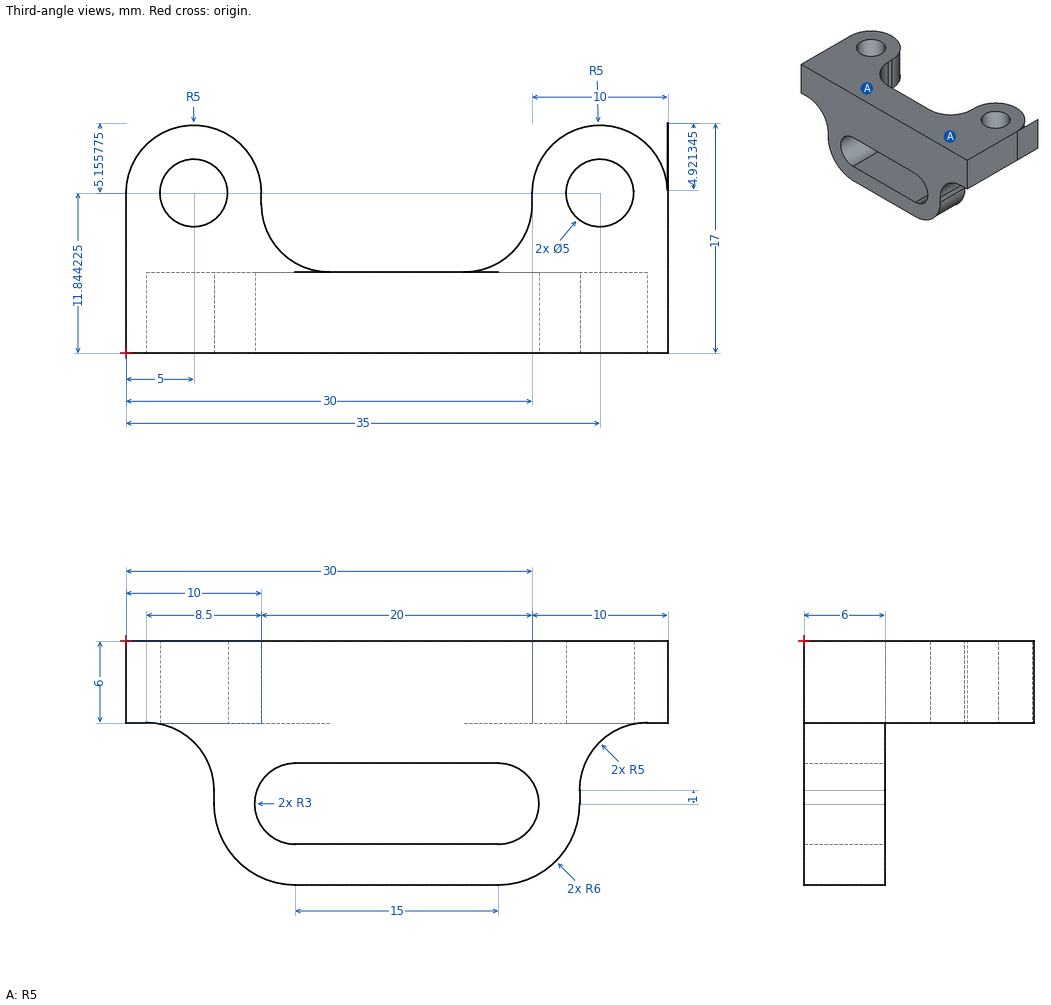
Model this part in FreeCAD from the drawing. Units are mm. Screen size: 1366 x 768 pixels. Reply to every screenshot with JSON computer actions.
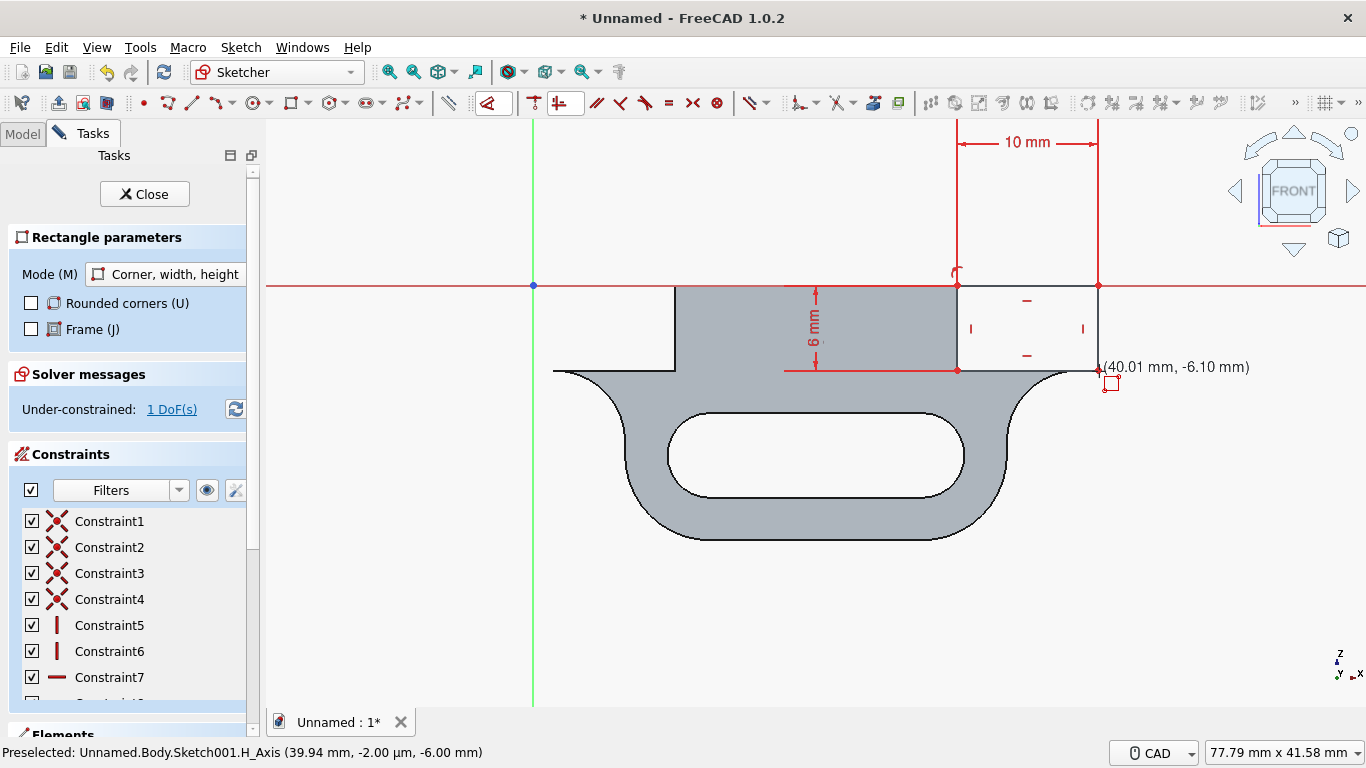
{"action": "left_click", "coordinate": [533, 286]}
{"action": "mouse_move", "coordinate": [675, 371]}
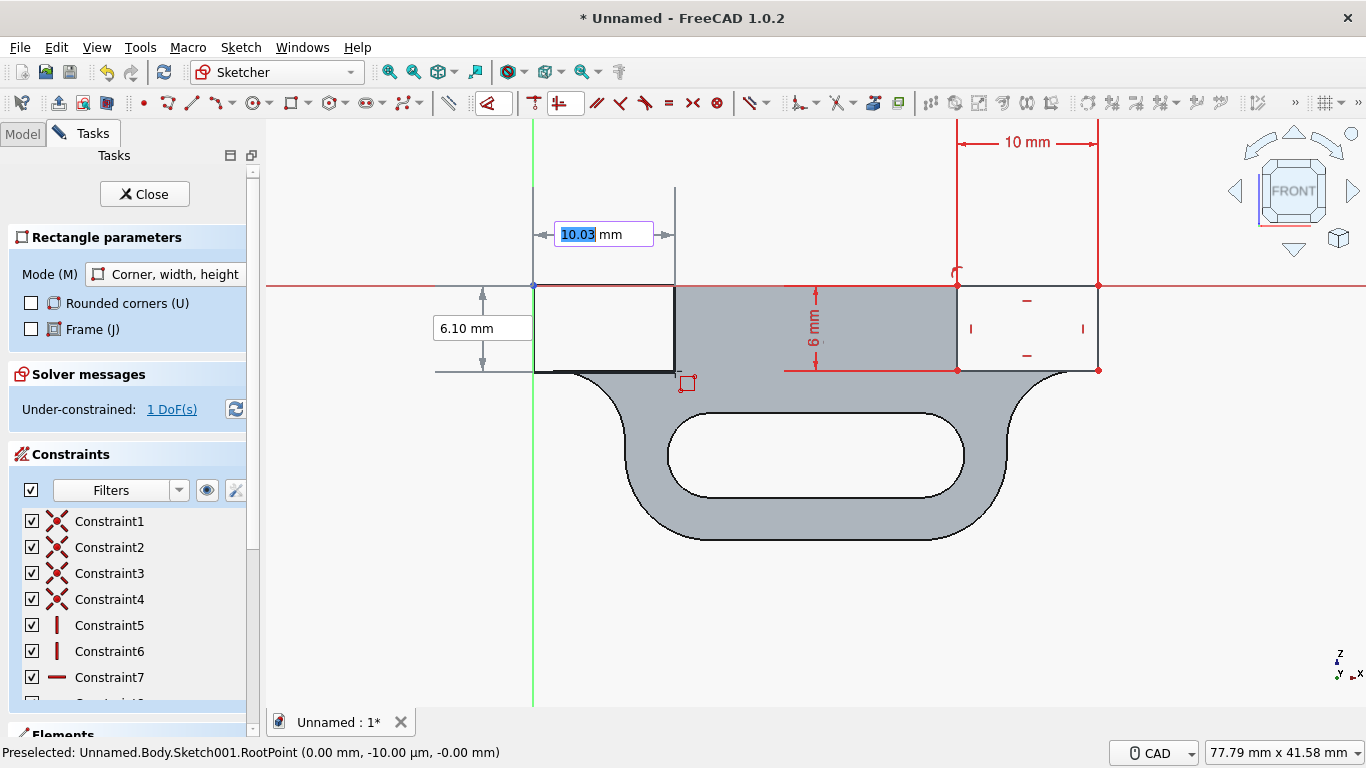
{"action": "type", "text": "10"}
{"action": "key", "text": "Tab"}
{"action": "type", "text": "6"}
{"action": "key", "text": "Return"}
{"action": "key", "text": "Escape"}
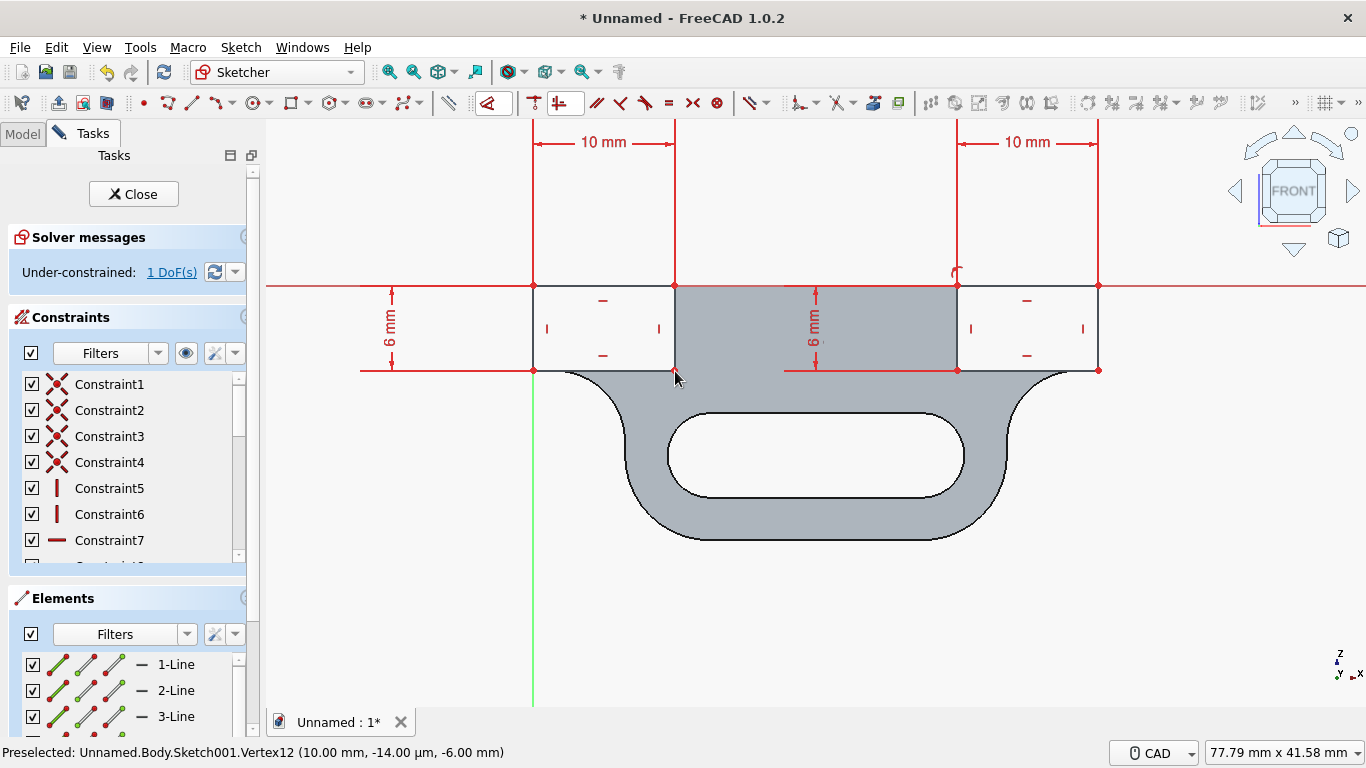
{"action": "left_click", "coordinate": [957, 286]}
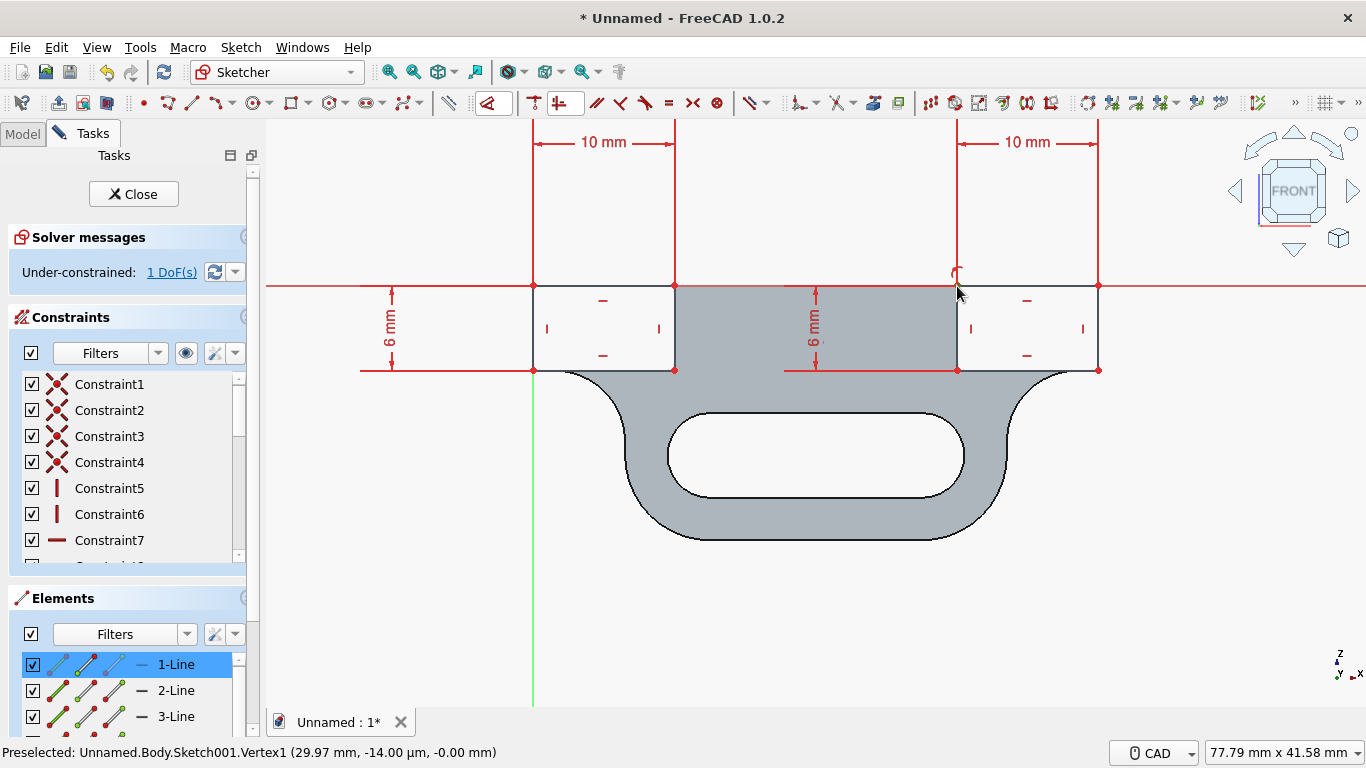
{"action": "key", "text": "l"}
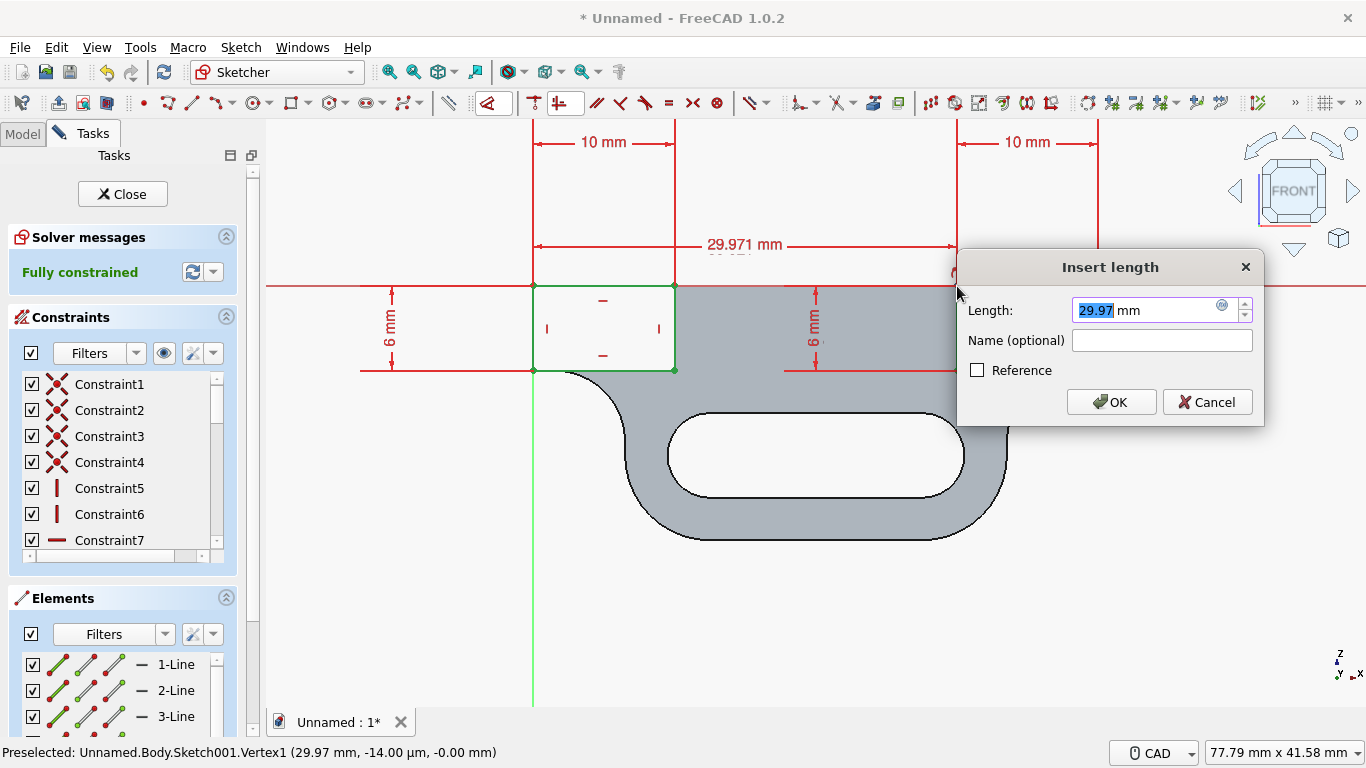
{"action": "type", "text": "30"}
{"action": "key", "text": "Return"}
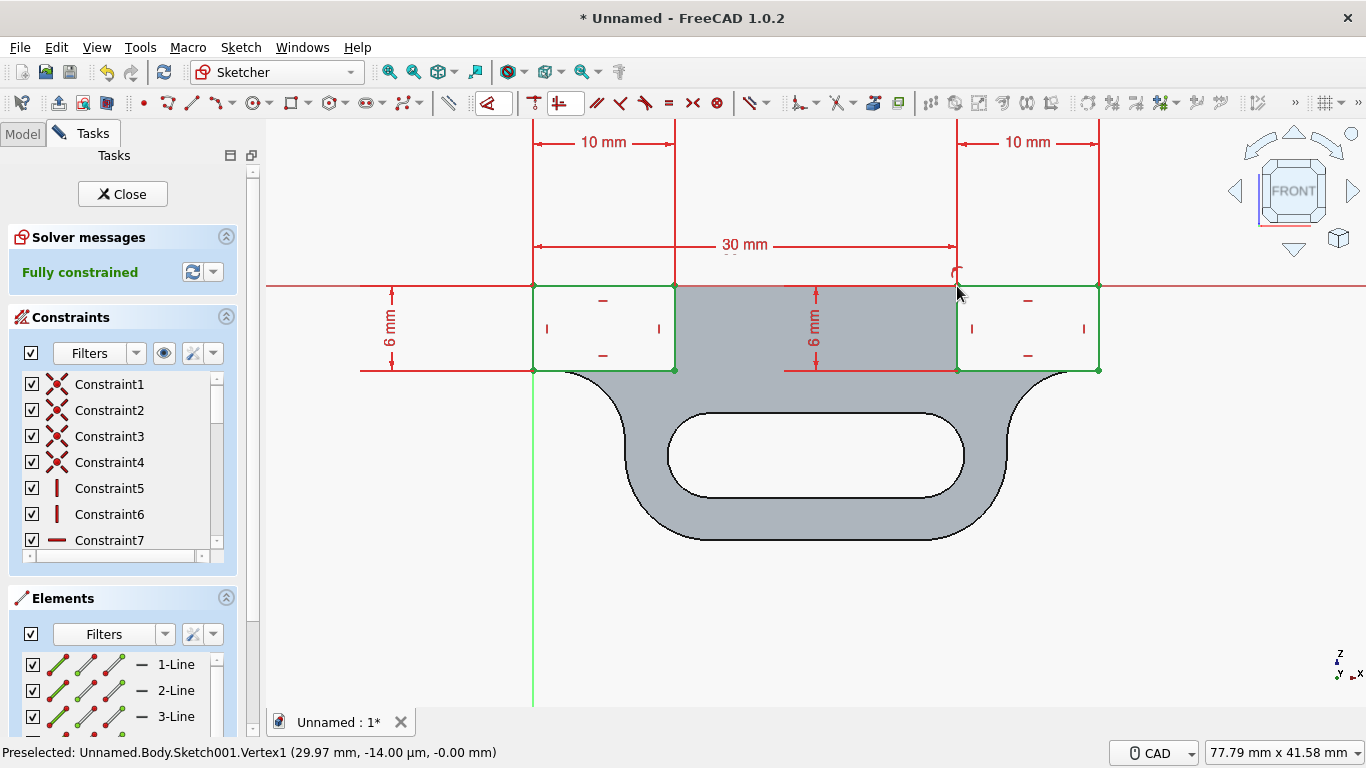
{"action": "left_click", "coordinate": [123, 194]}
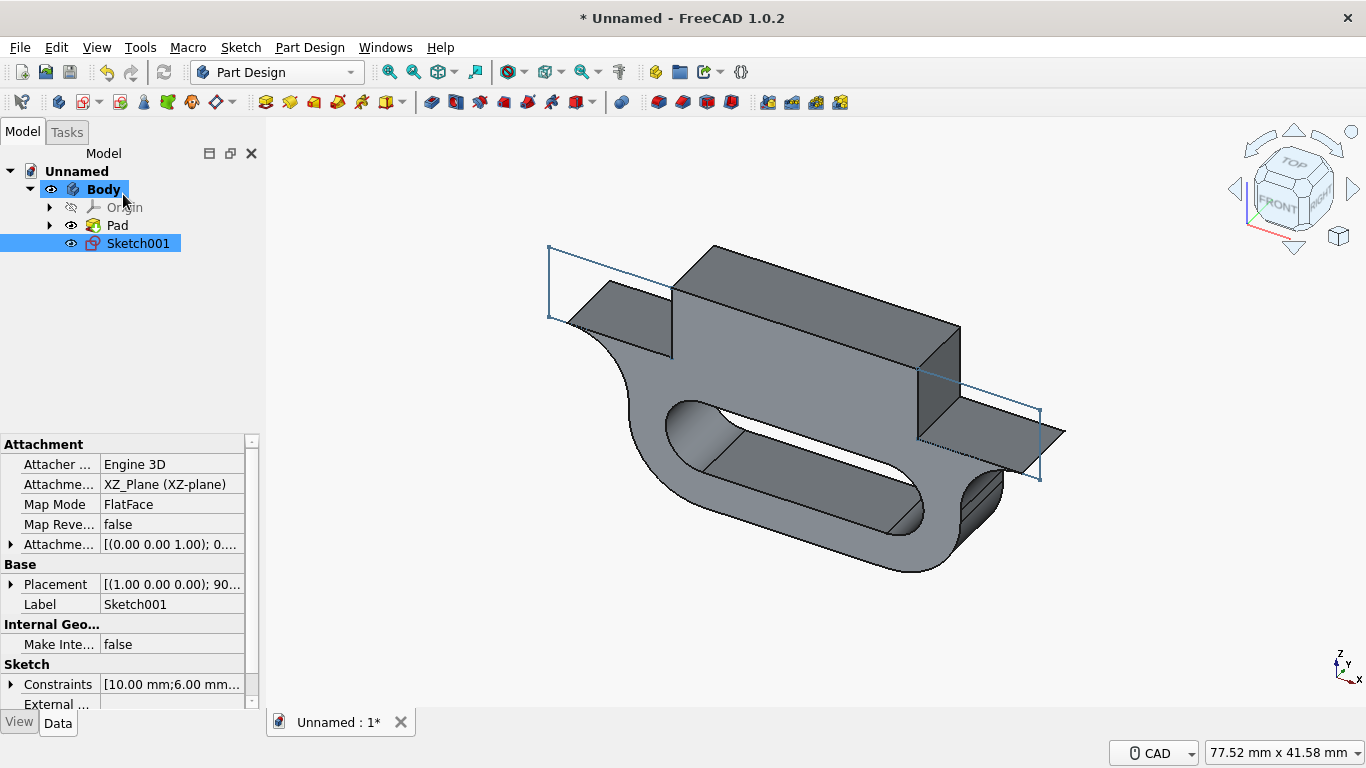
{"action": "left_click", "coordinate": [266, 102]}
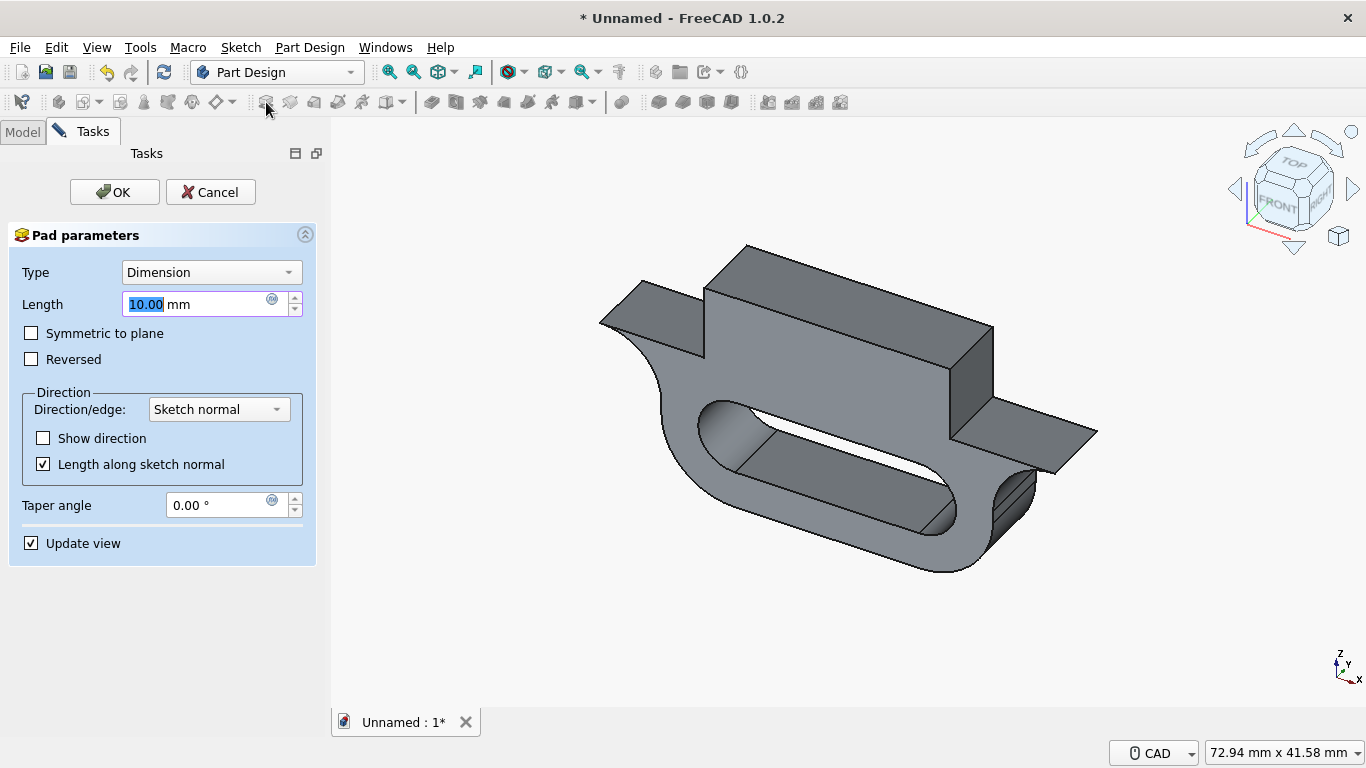
{"action": "type", "text": "17"}
{"action": "key", "text": "Tab"}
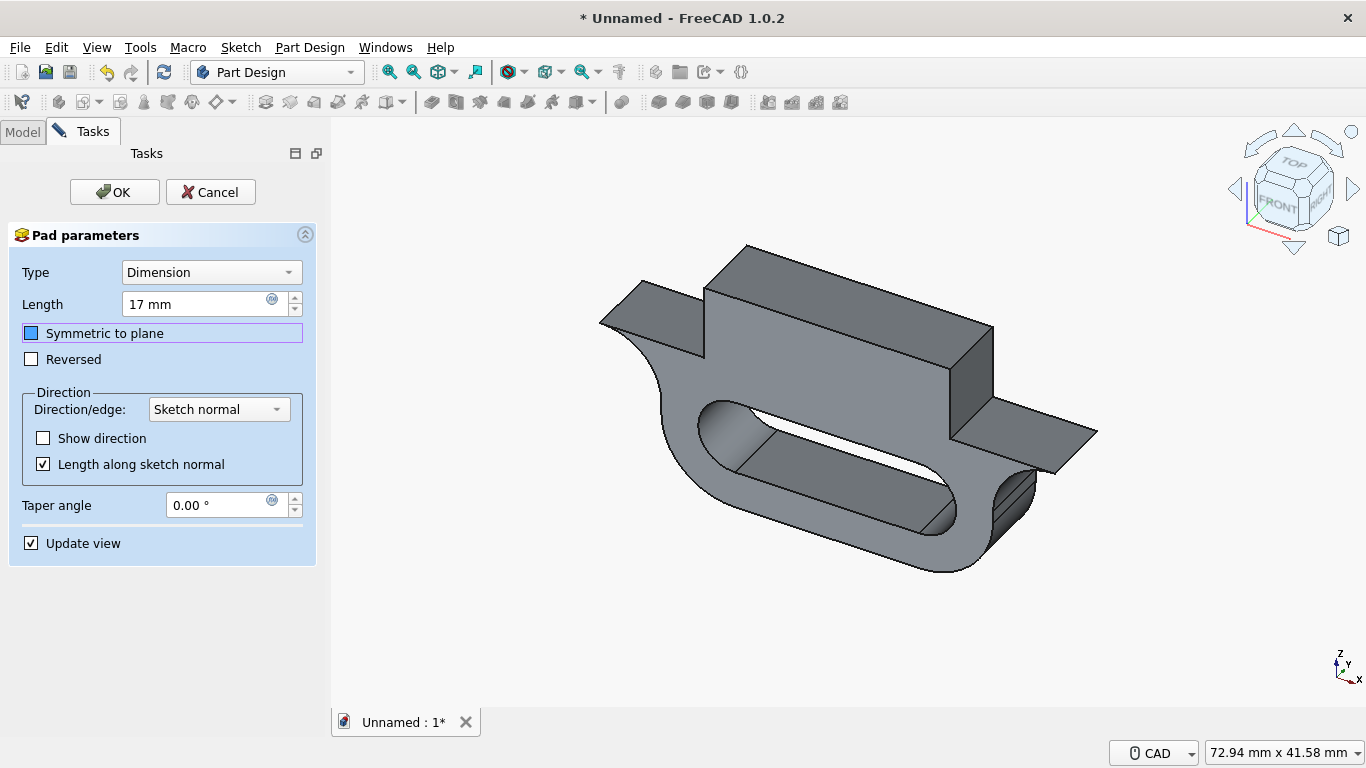
{"action": "left_click", "coordinate": [30, 359]}